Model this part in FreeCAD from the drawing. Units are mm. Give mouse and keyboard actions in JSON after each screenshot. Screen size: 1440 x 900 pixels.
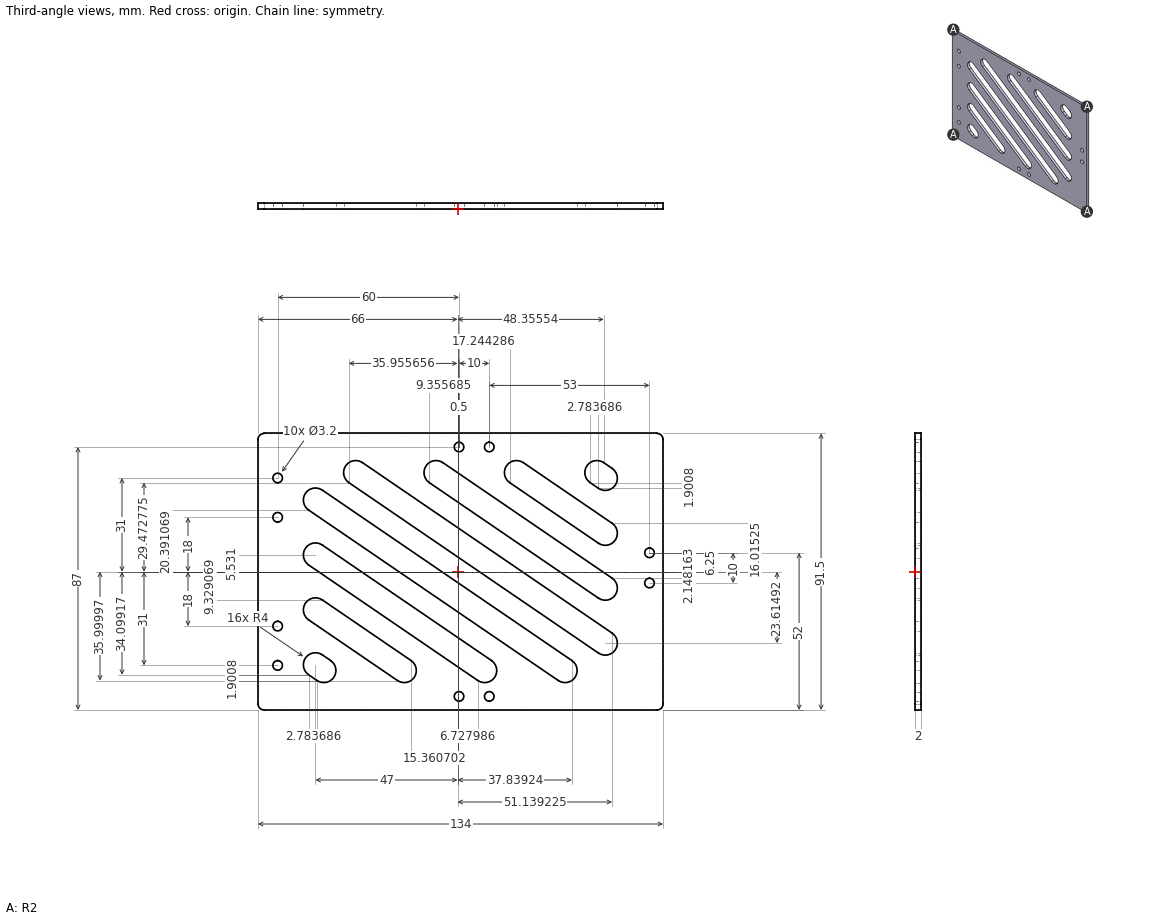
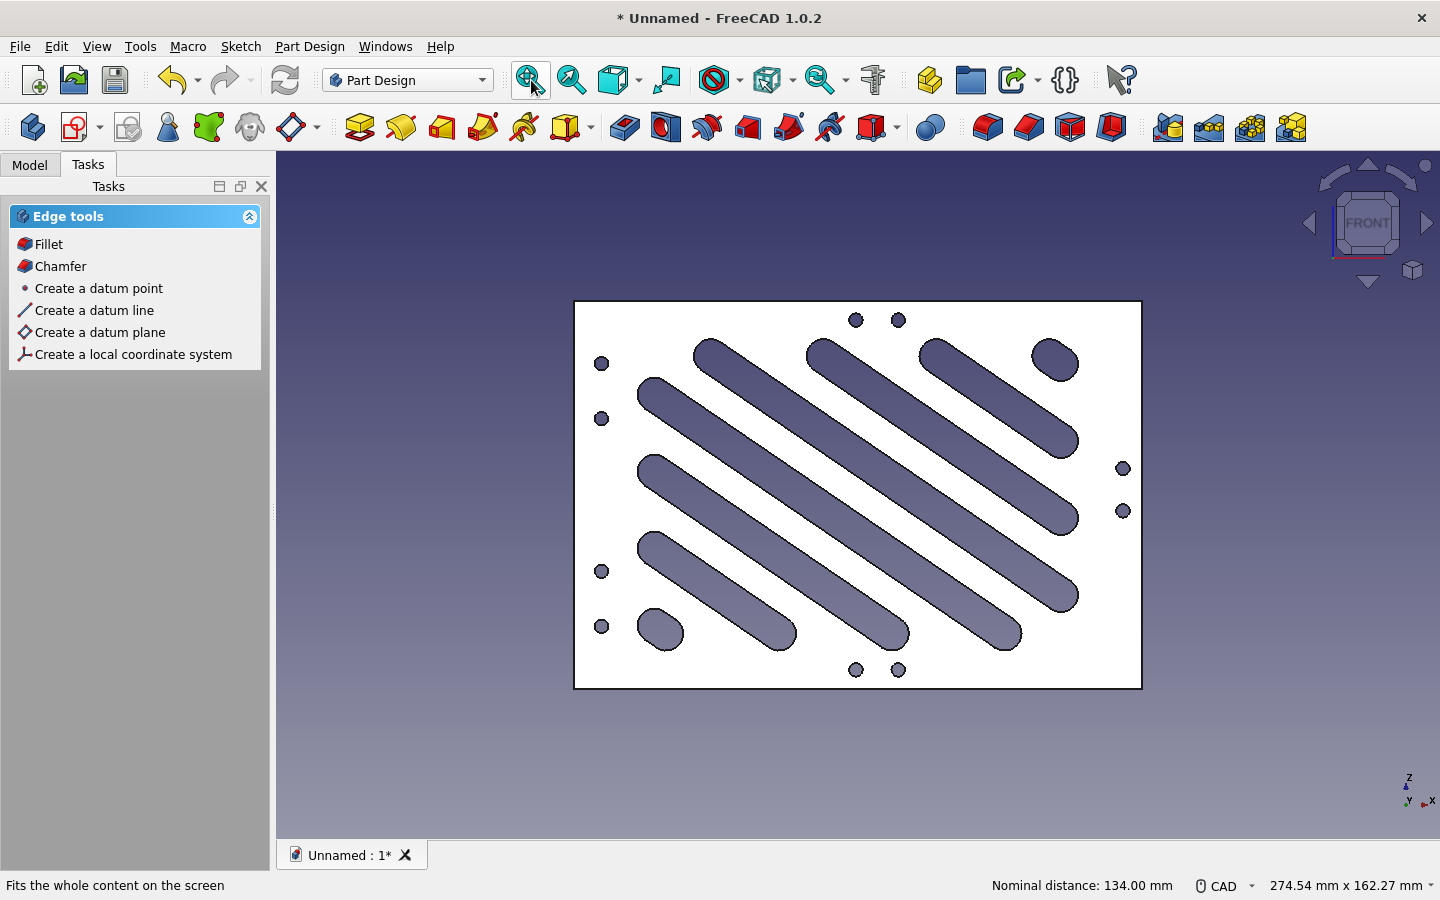
{"action": "key", "text": "3"}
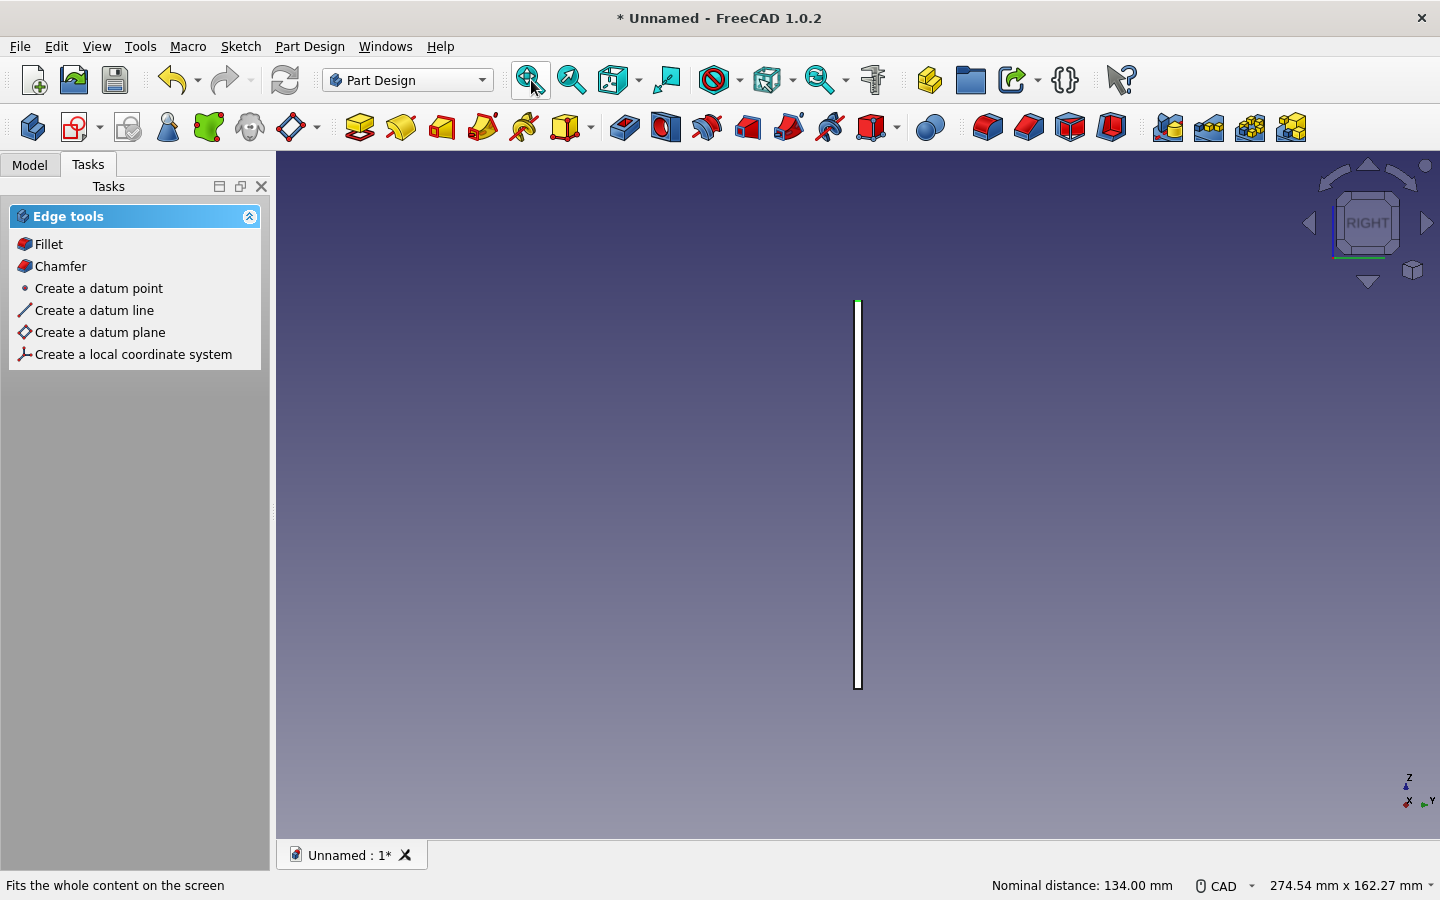
{"action": "scroll", "coordinate": [858, 688], "scroll_direction": "up", "scroll_amount": 8}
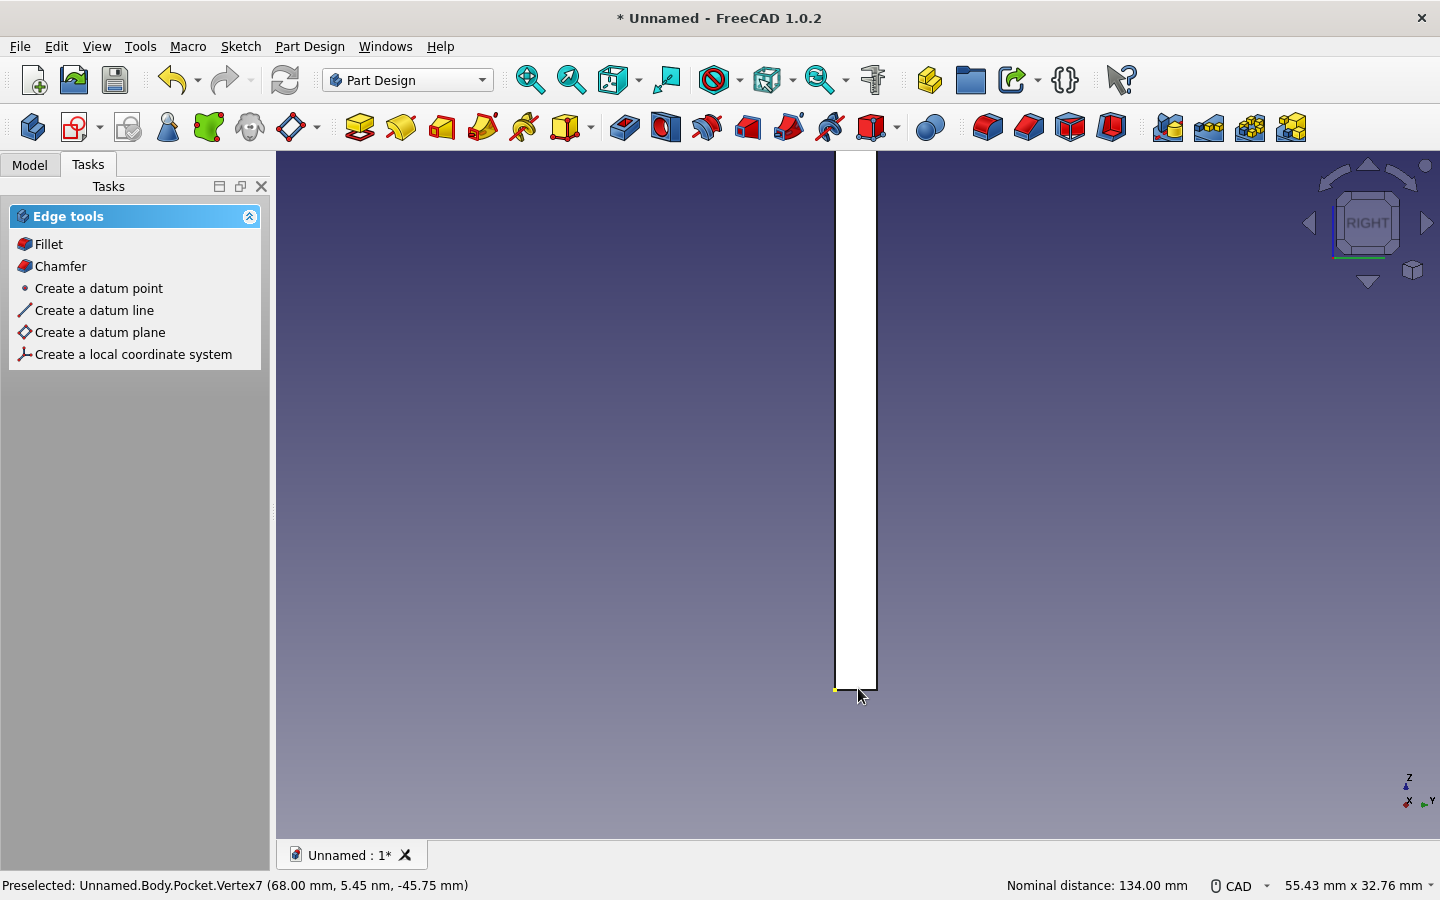
{"action": "left_click", "coordinate": [856, 689], "text": "ctrl"}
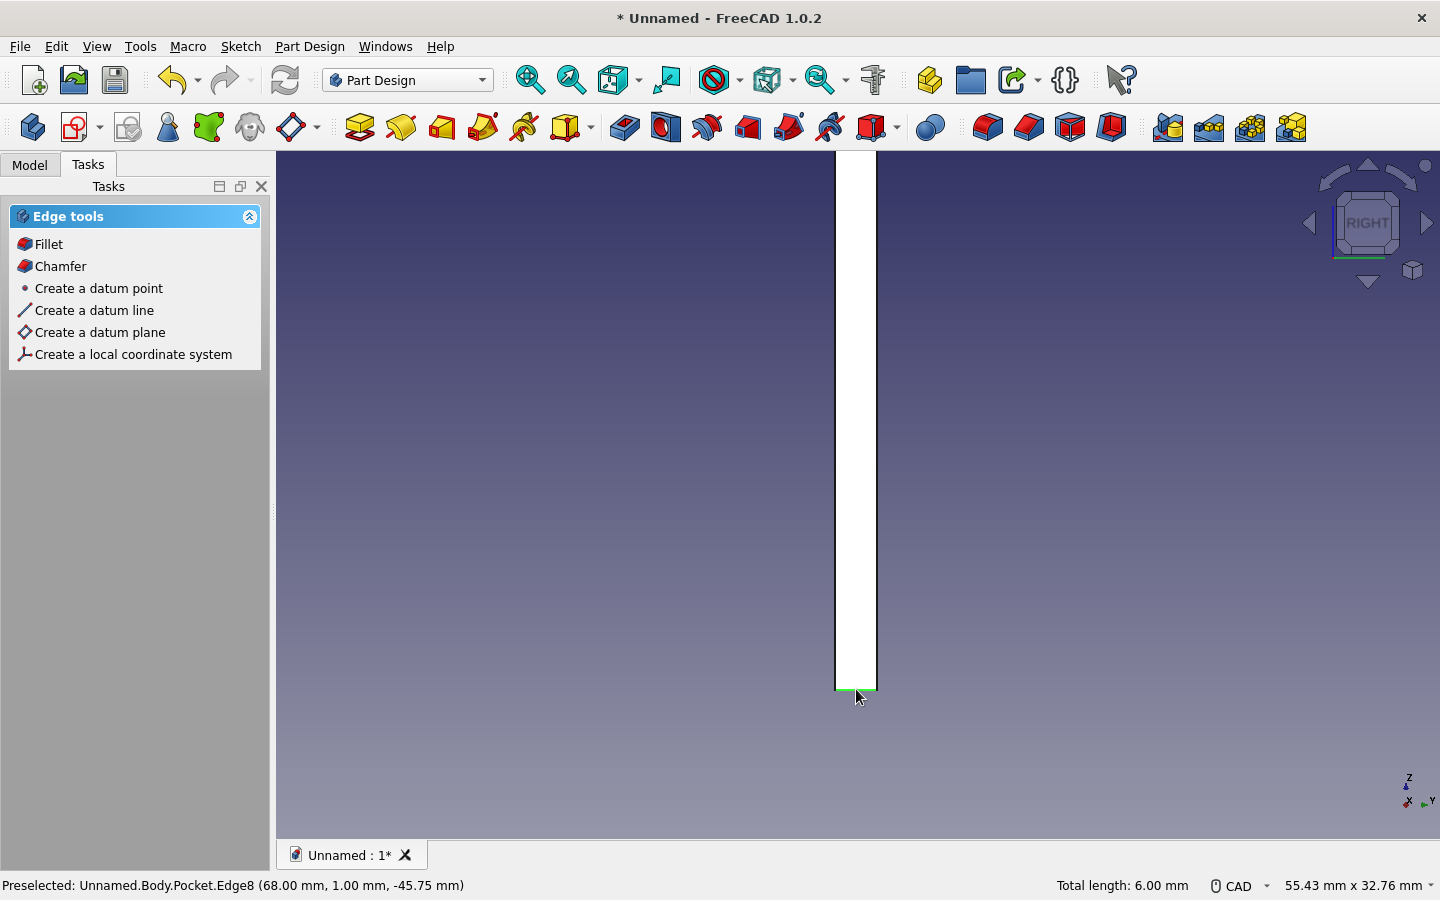
{"action": "left_click", "coordinate": [531, 80]}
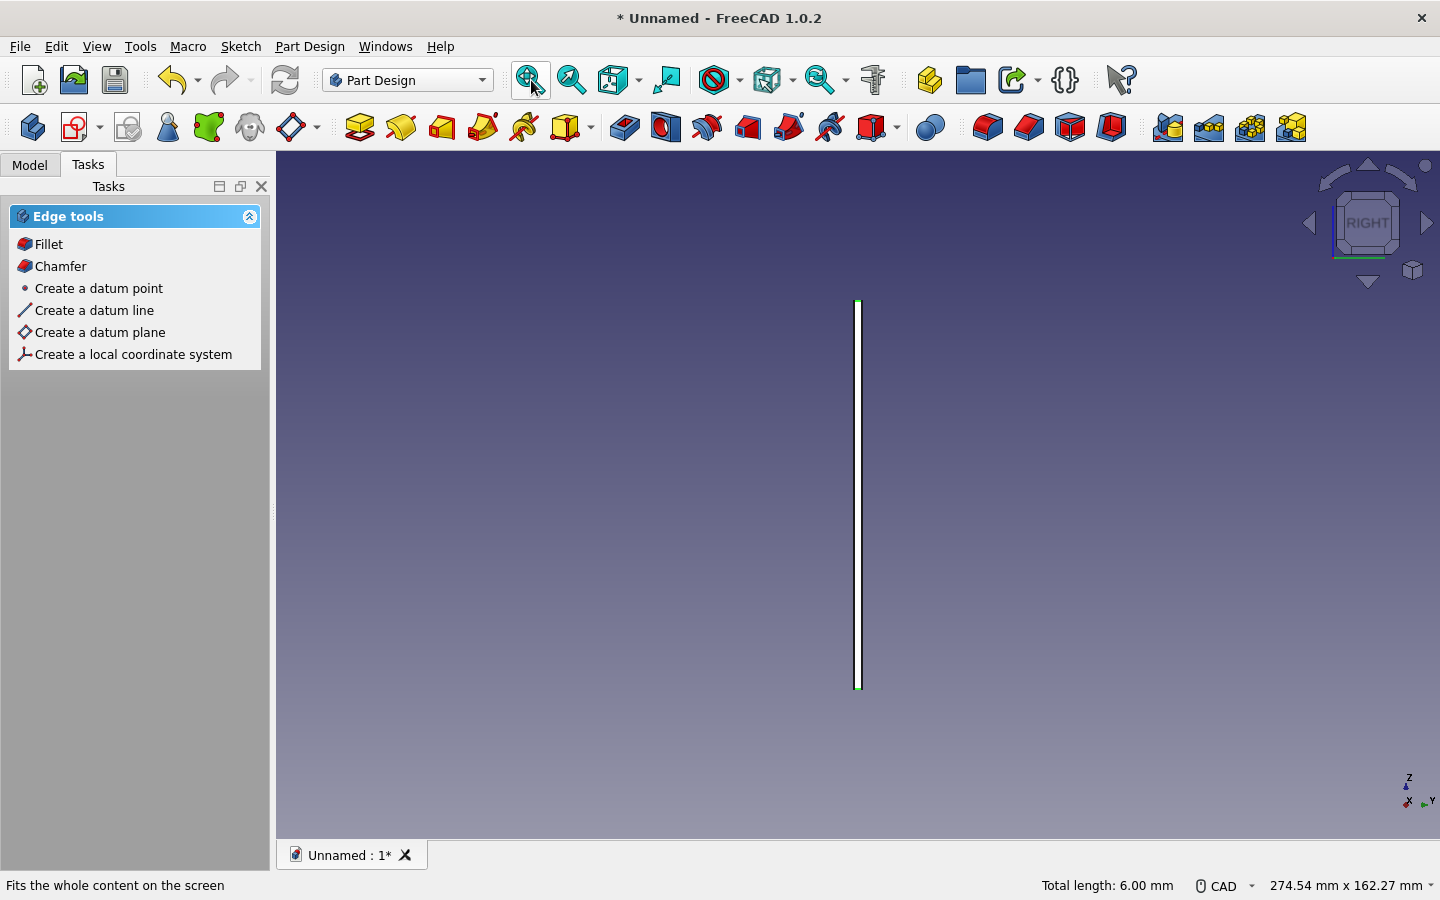
{"action": "key", "text": "5"}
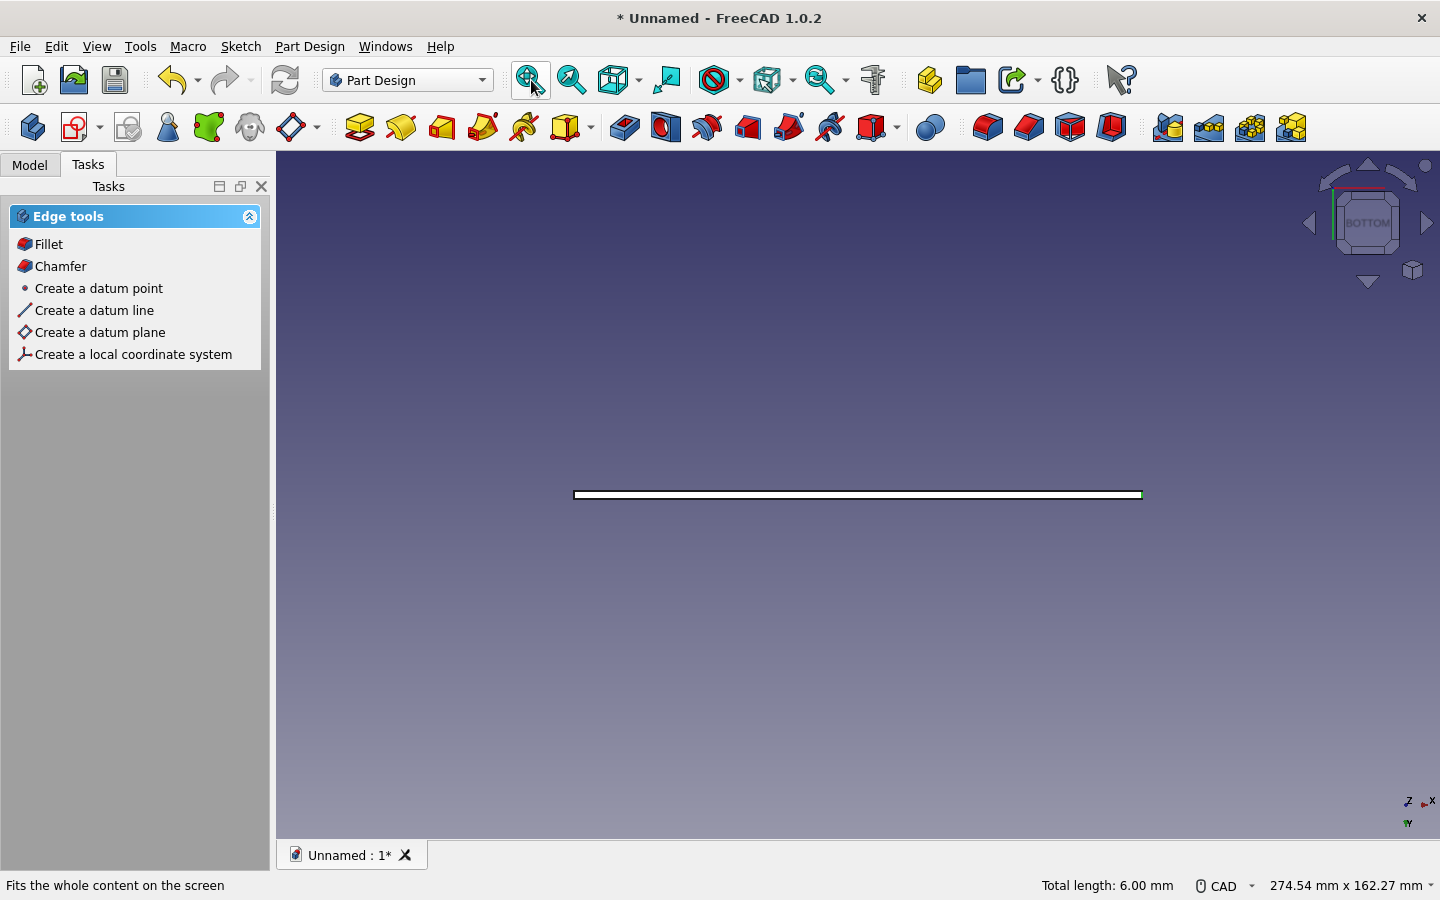
{"action": "left_click", "coordinate": [574, 496], "text": "ctrl"}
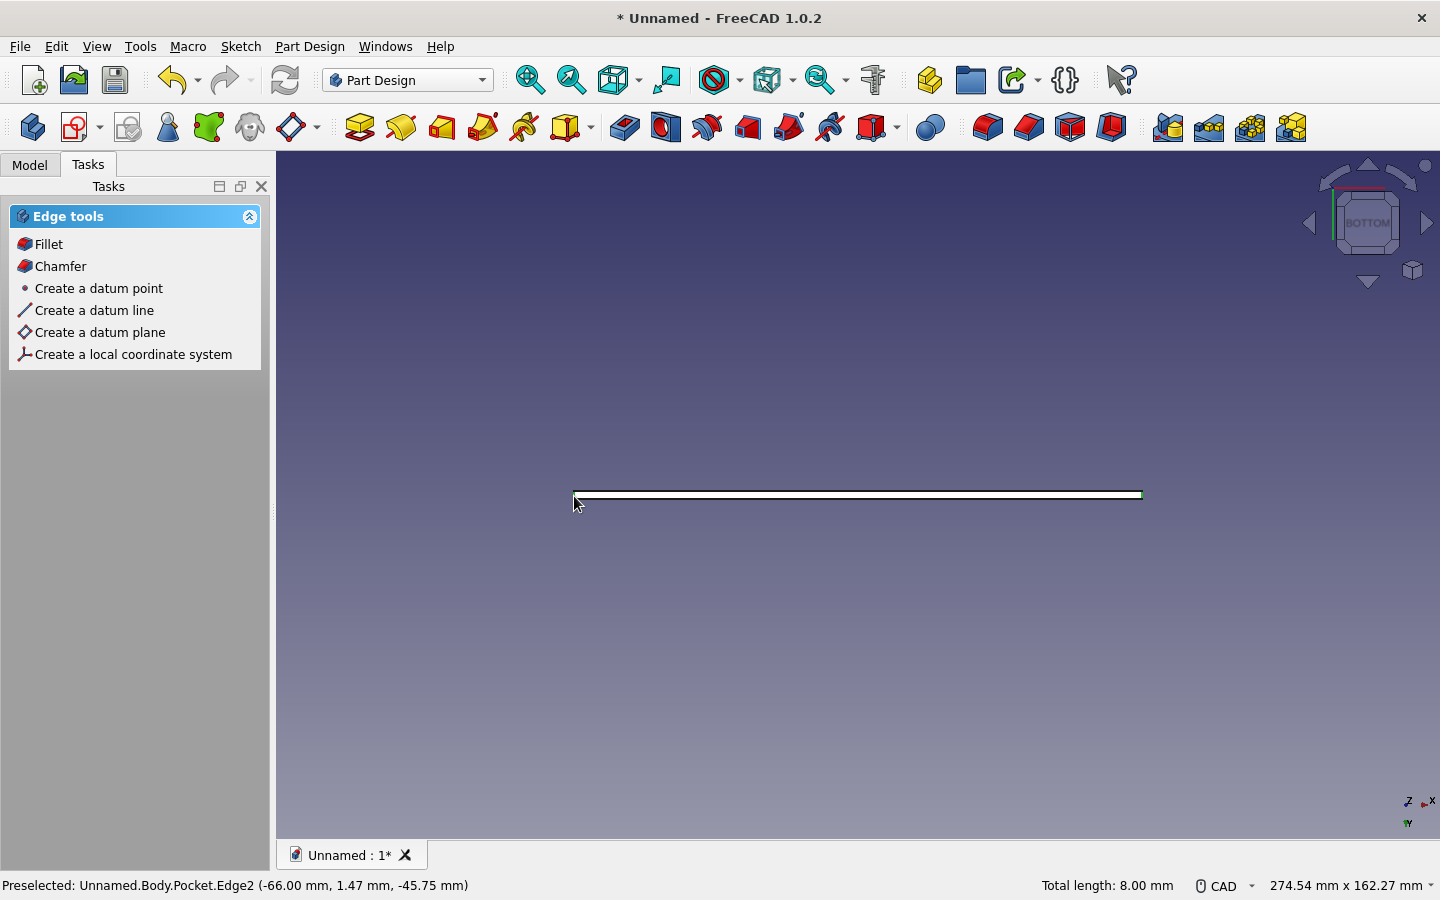
{"action": "left_click", "coordinate": [988, 128]}